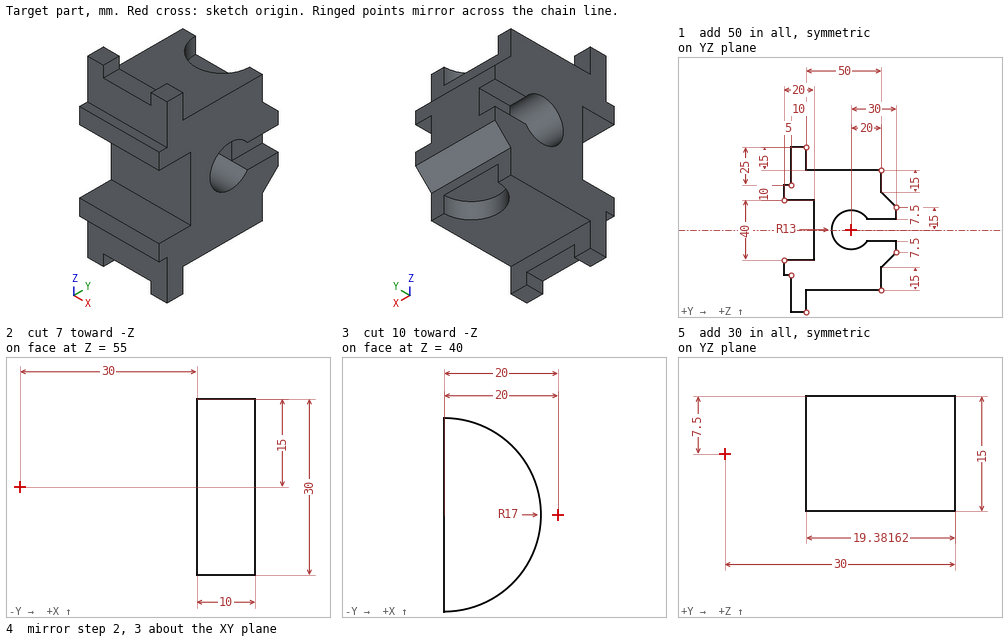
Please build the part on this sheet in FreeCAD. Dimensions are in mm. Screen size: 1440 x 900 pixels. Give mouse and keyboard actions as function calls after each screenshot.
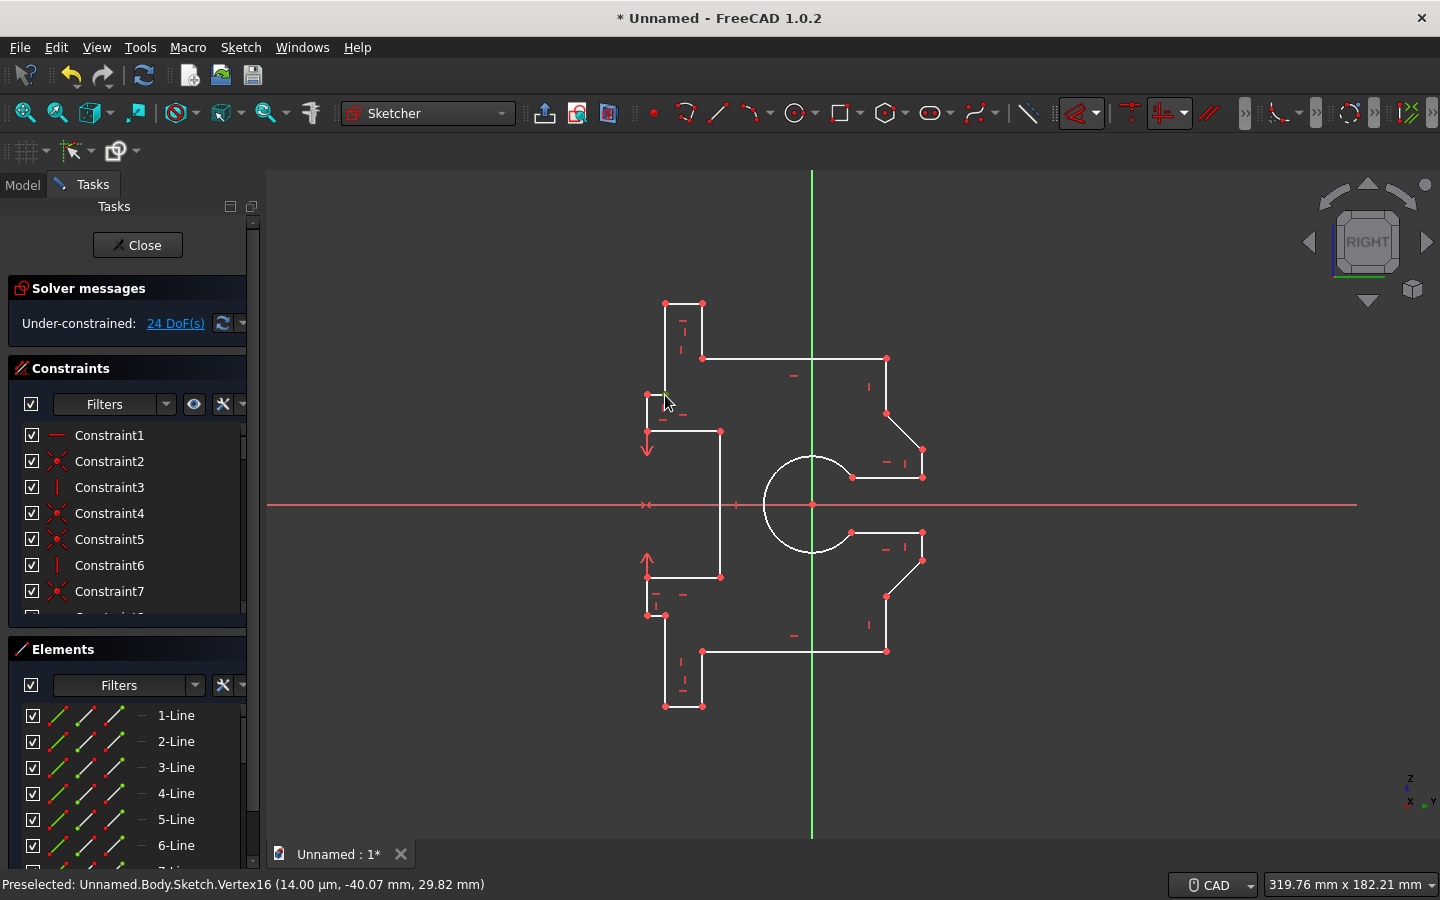
click(665, 616)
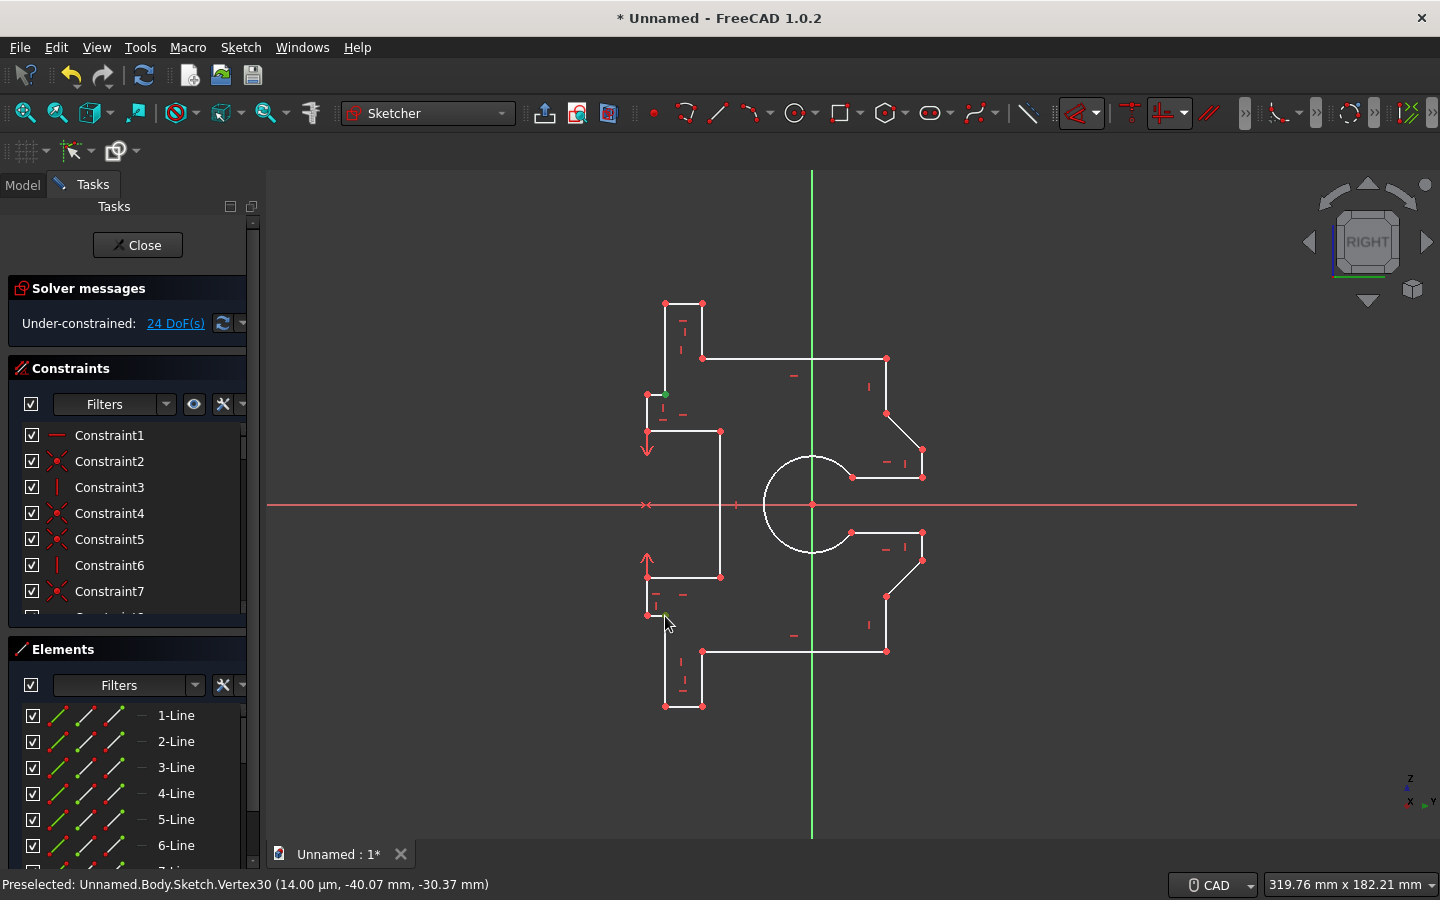
click(364, 504)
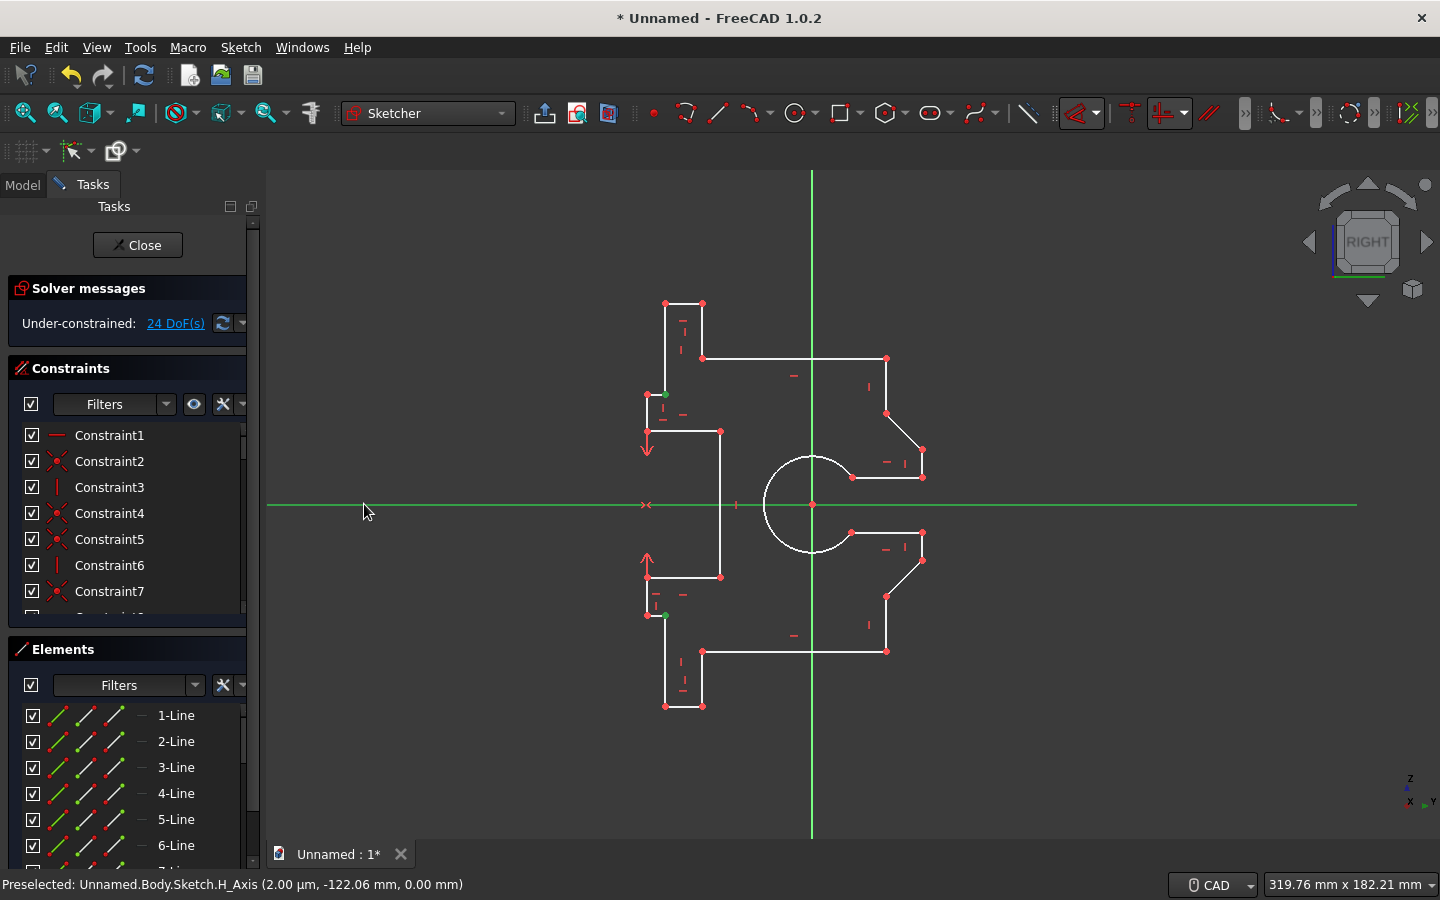
key(s)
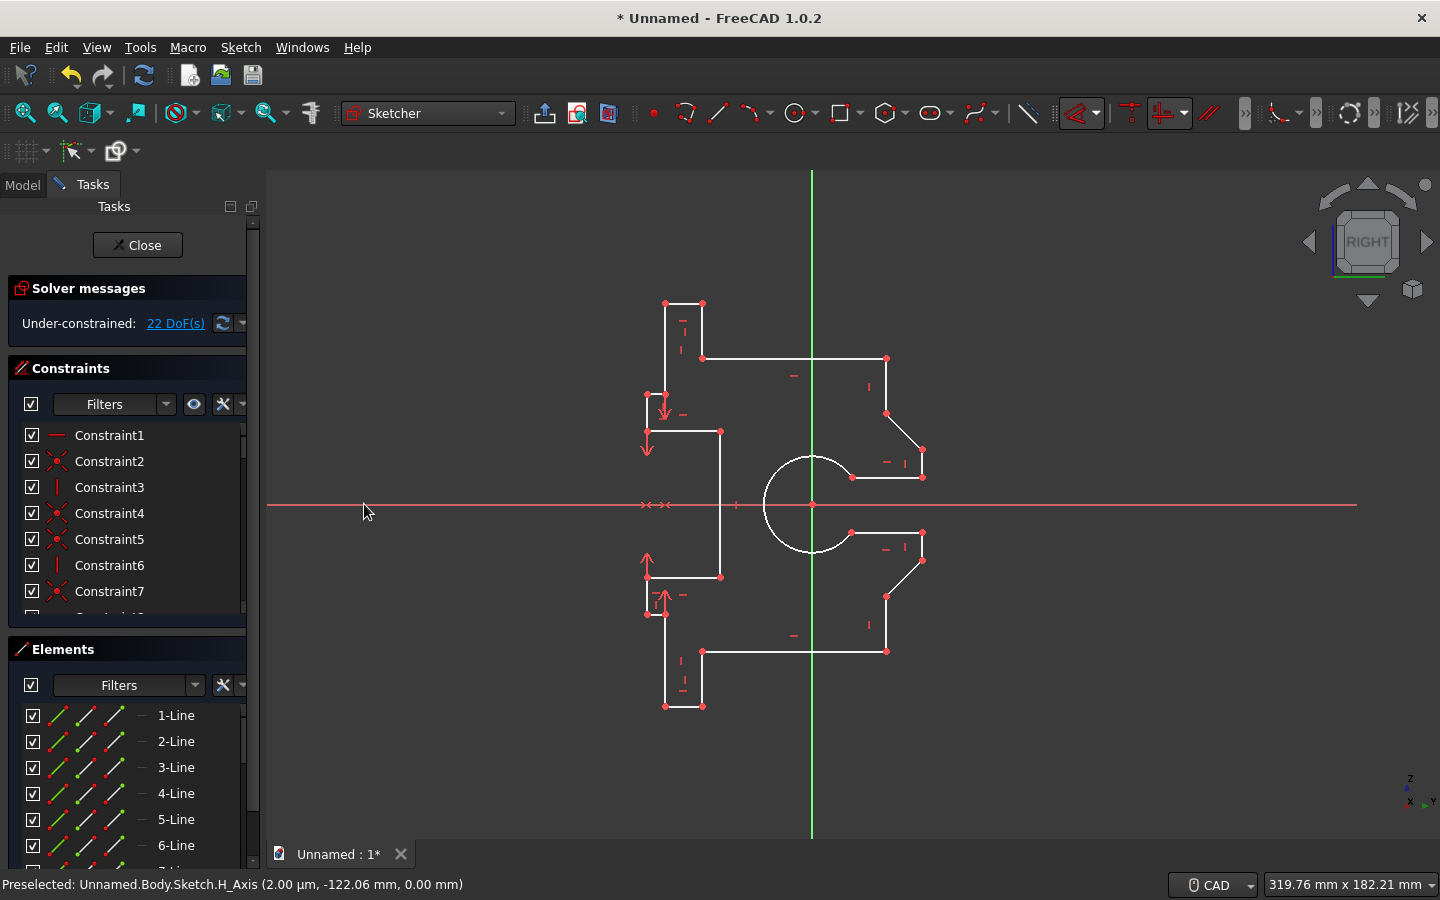
click(702, 304)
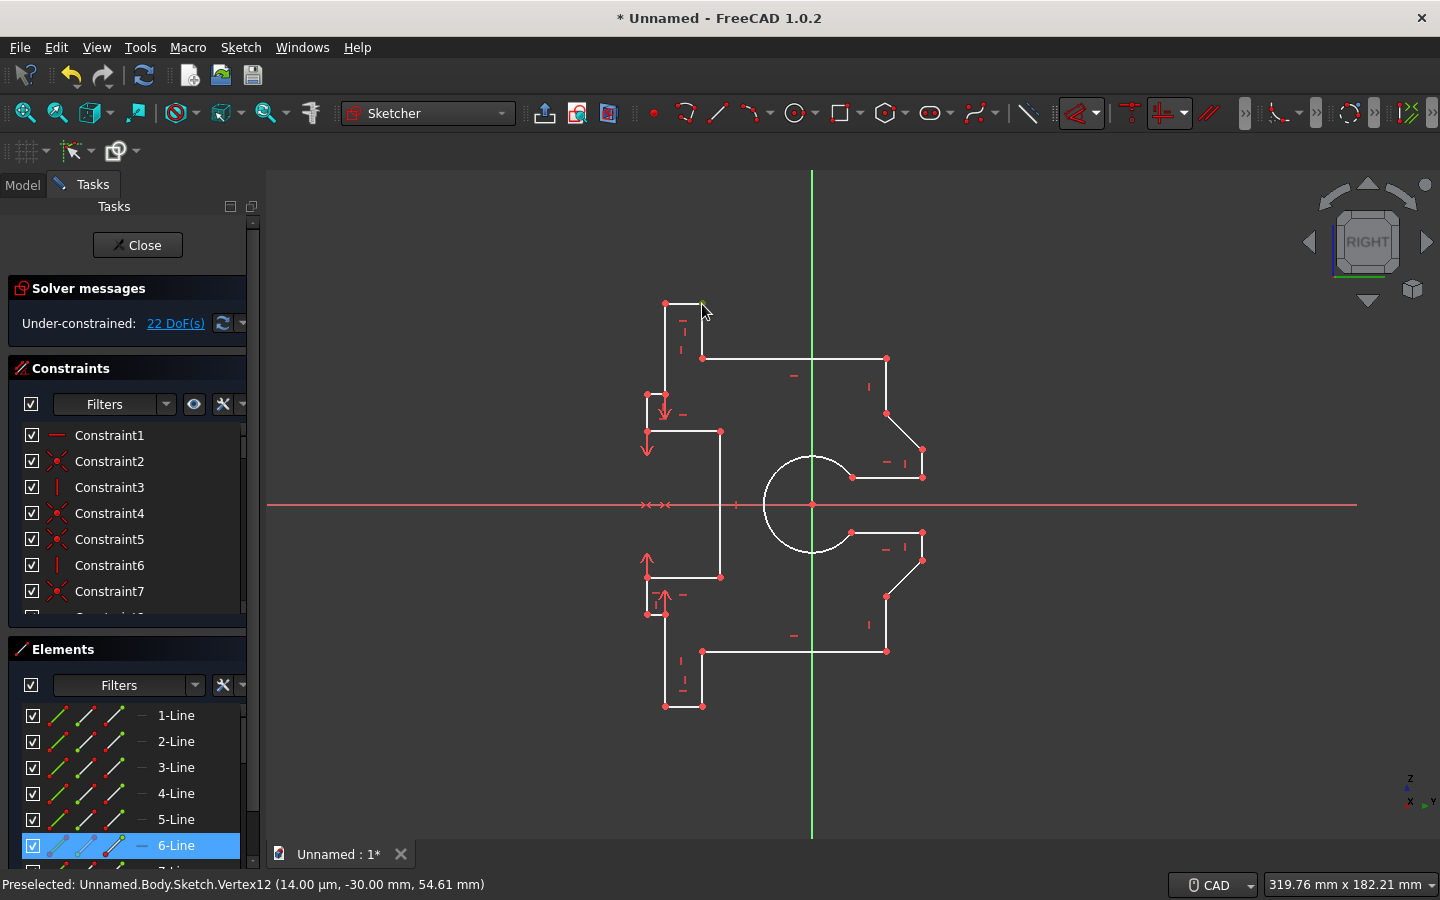
click(702, 707)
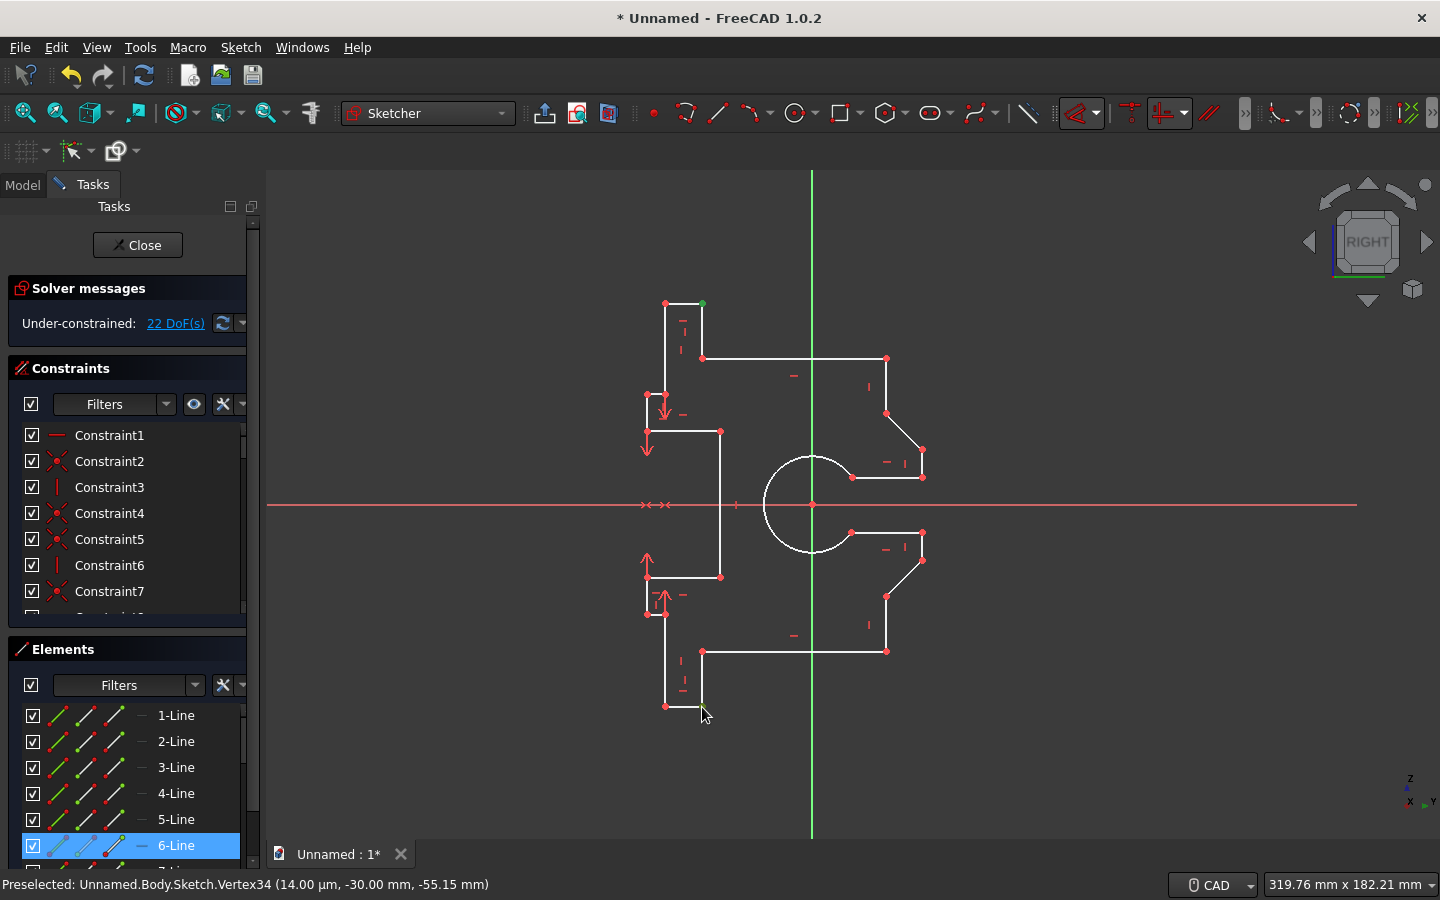
click(364, 504)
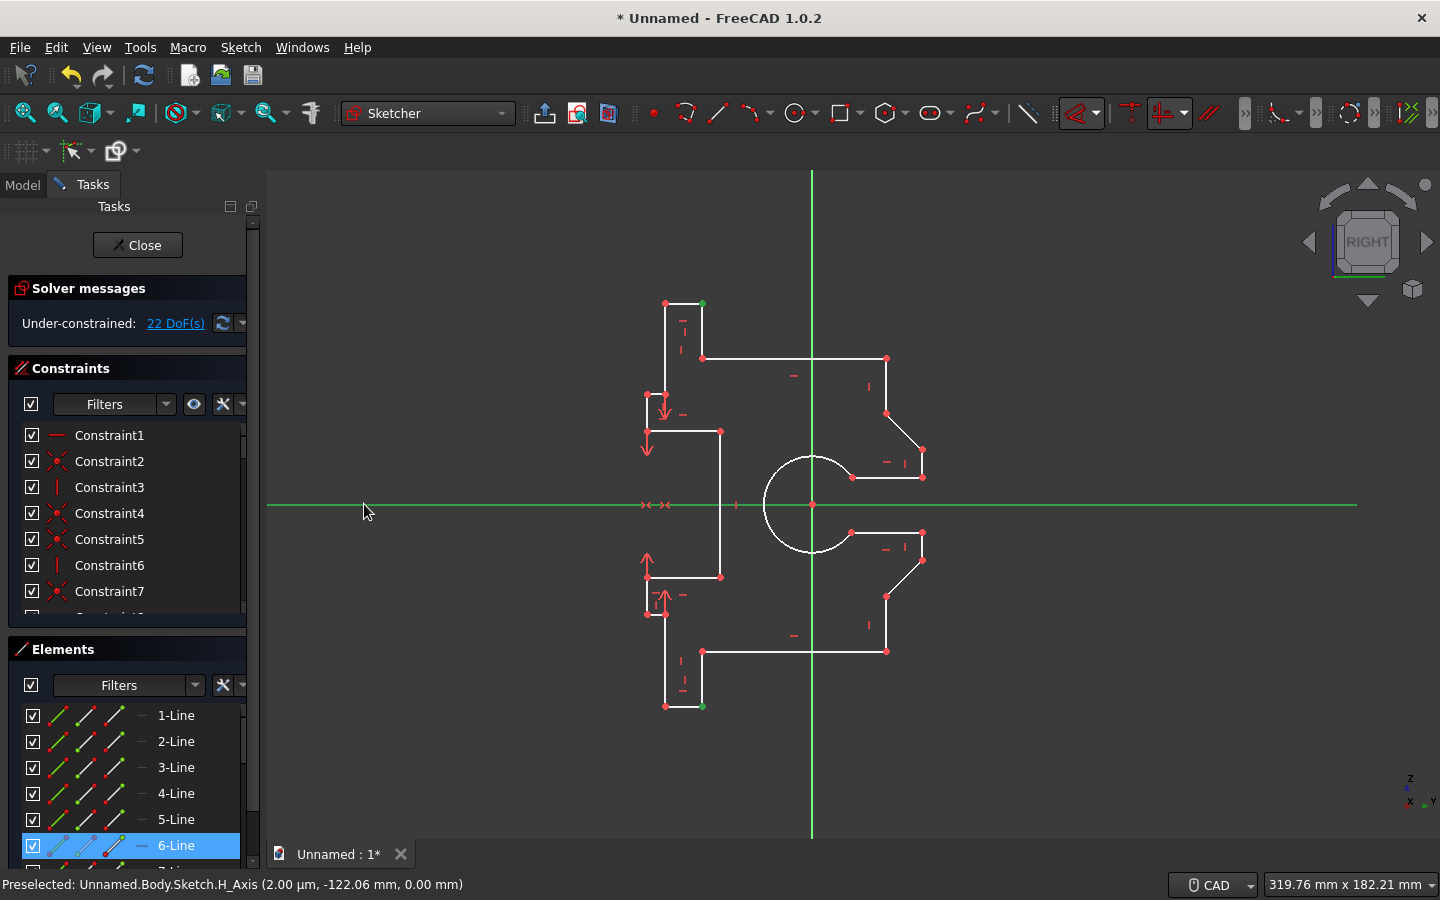
key(s)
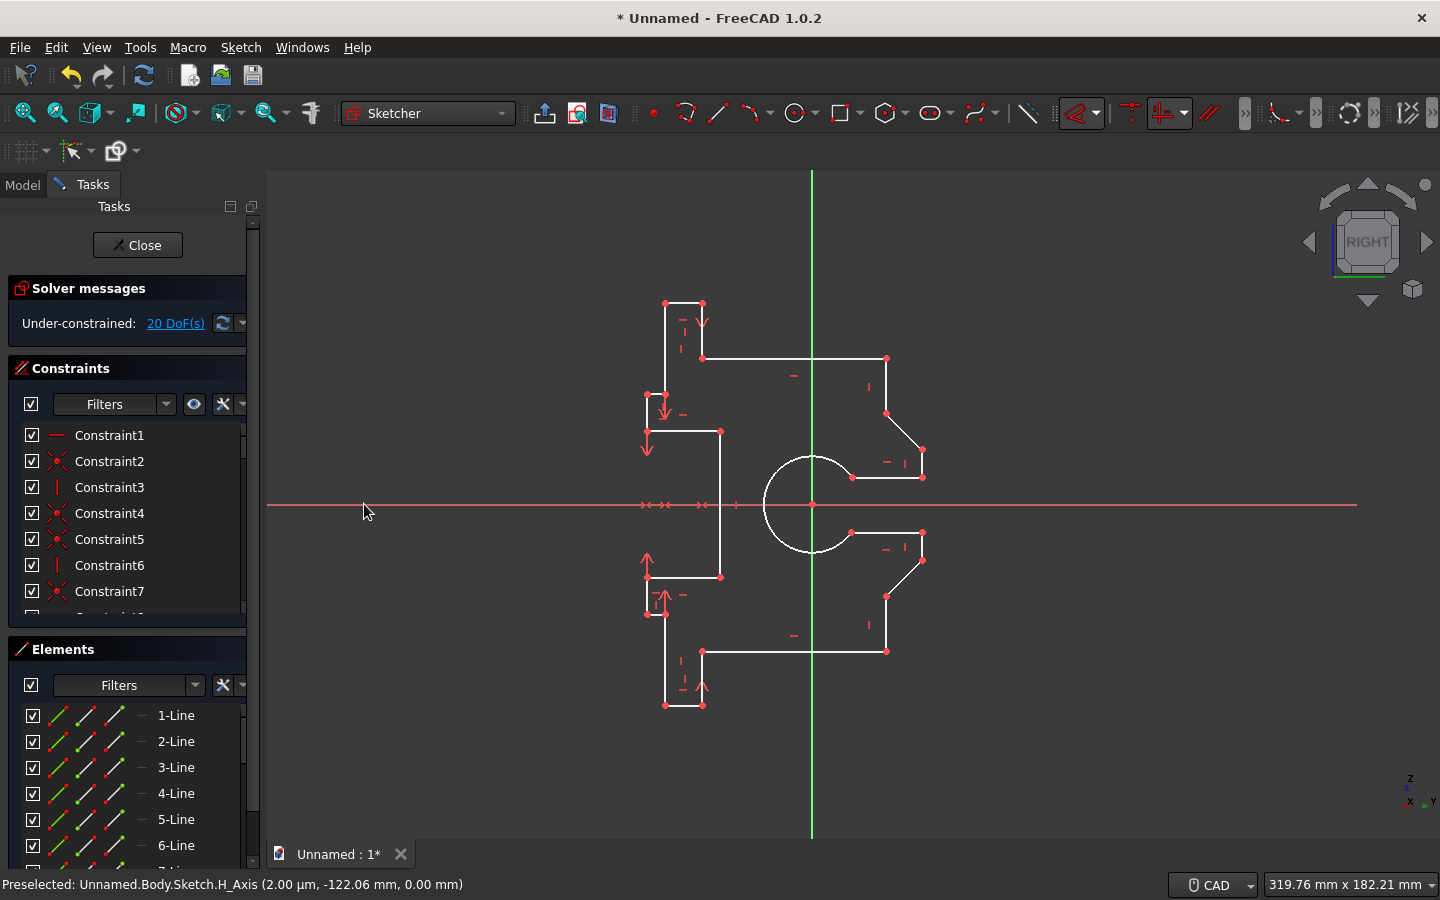
click(886, 359)